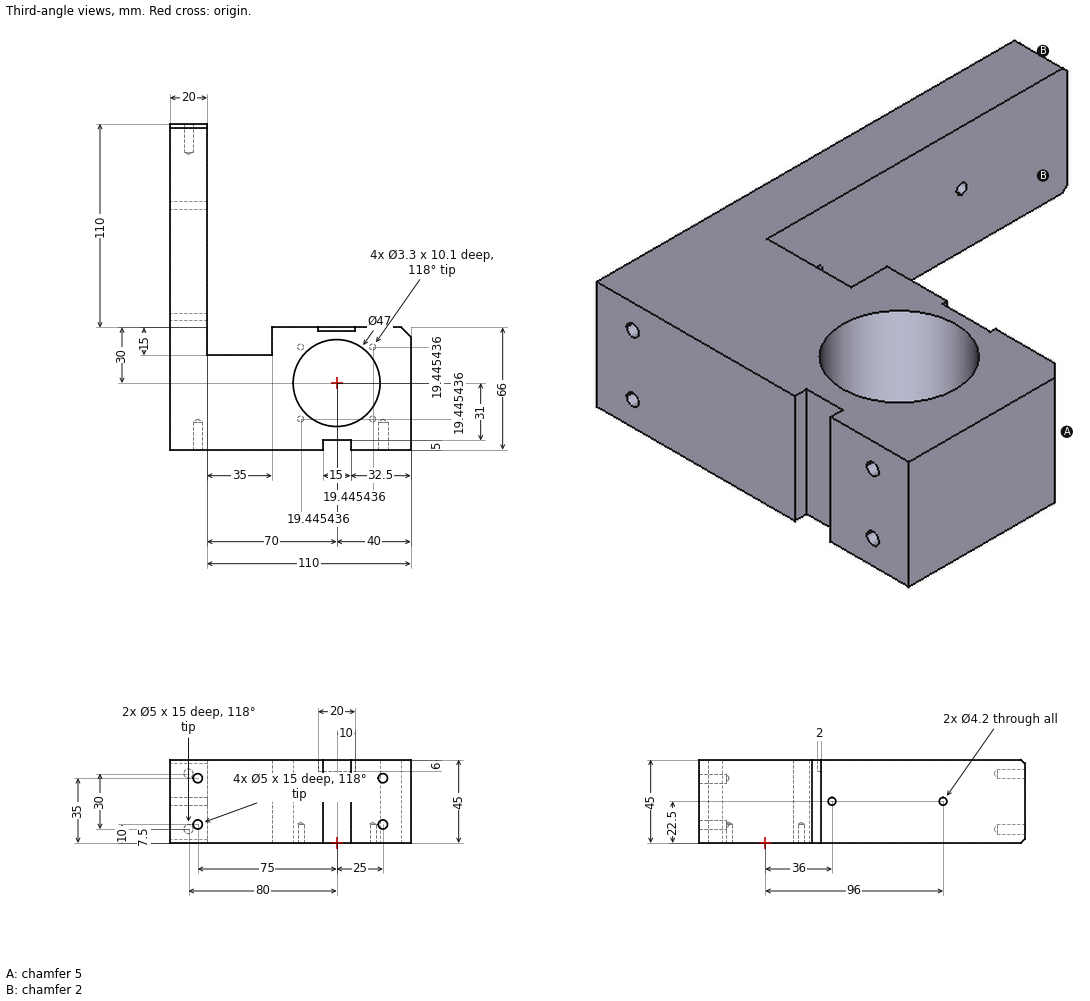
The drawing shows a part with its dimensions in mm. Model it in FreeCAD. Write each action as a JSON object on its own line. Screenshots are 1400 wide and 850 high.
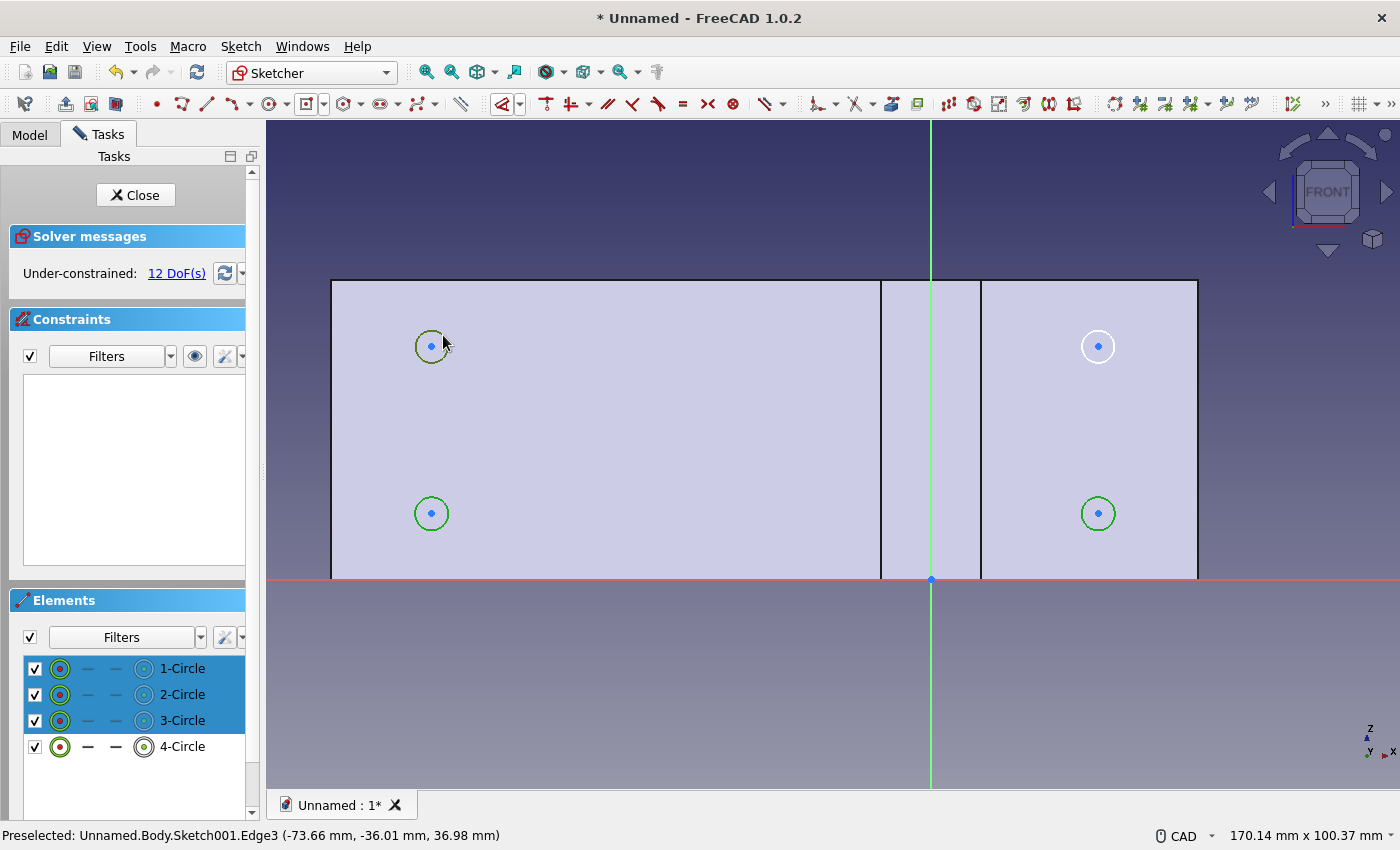
{"action": "left_click", "coordinate": [1110, 335]}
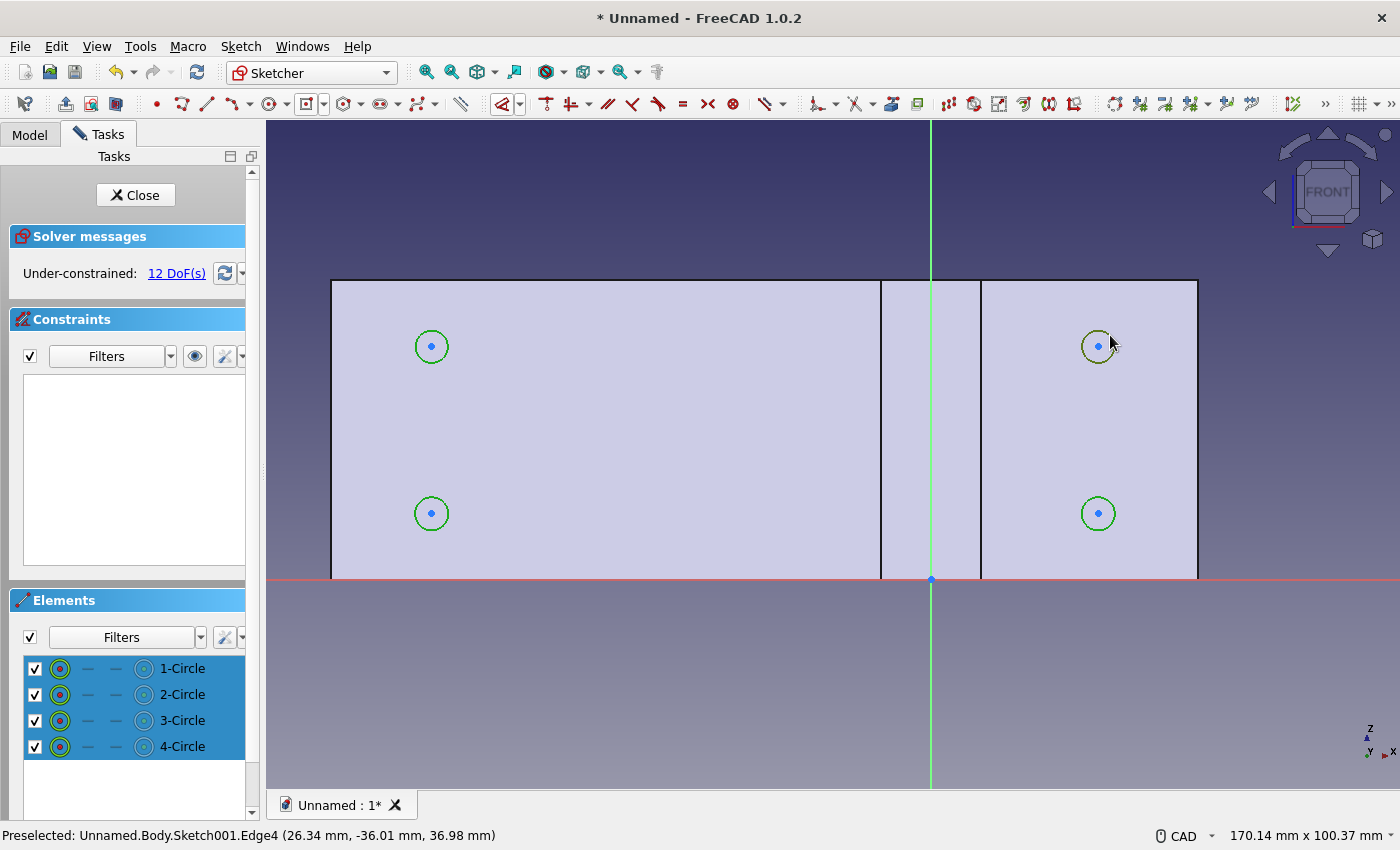
{"action": "key", "text": "e"}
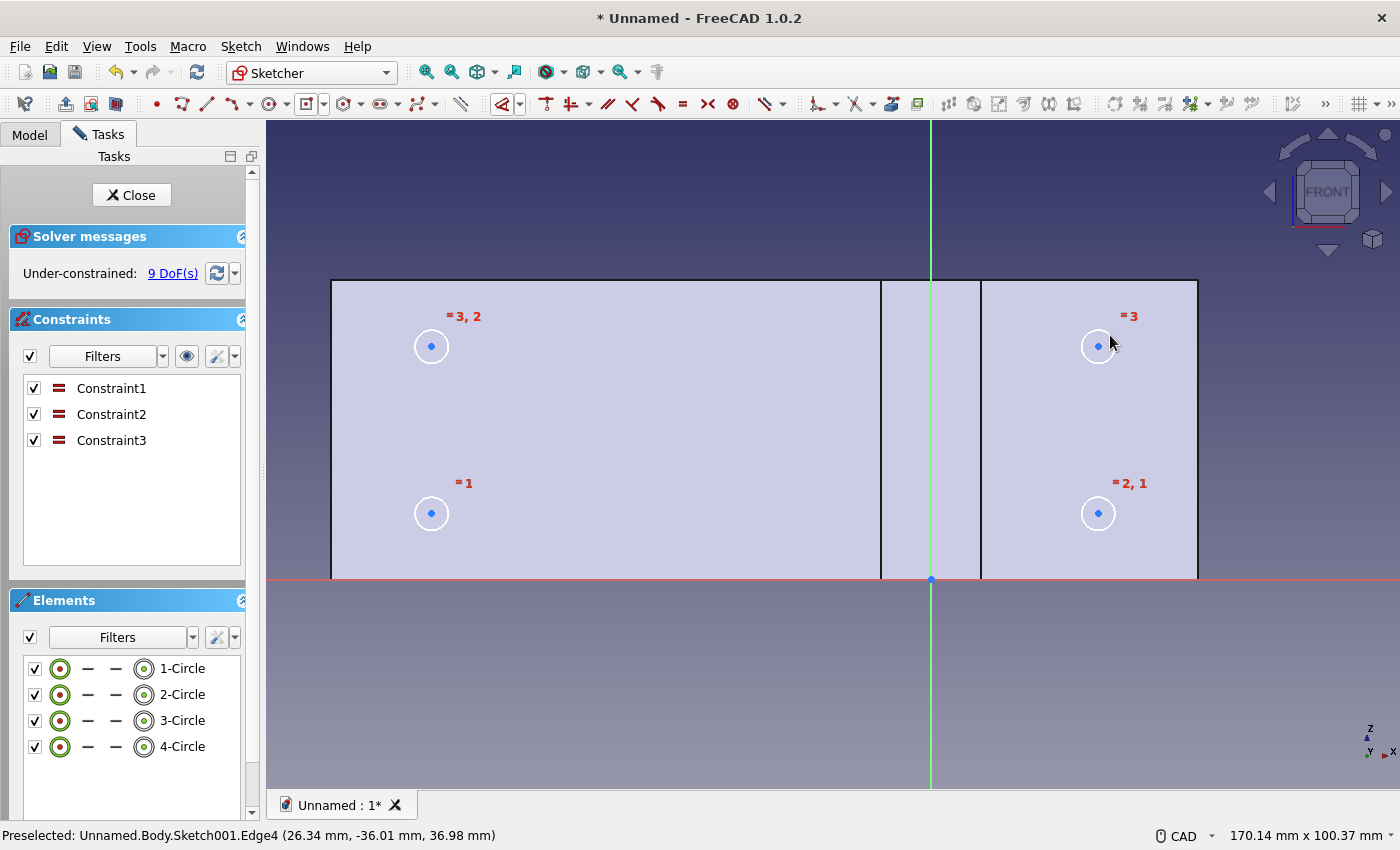
{"action": "left_click", "coordinate": [432, 514]}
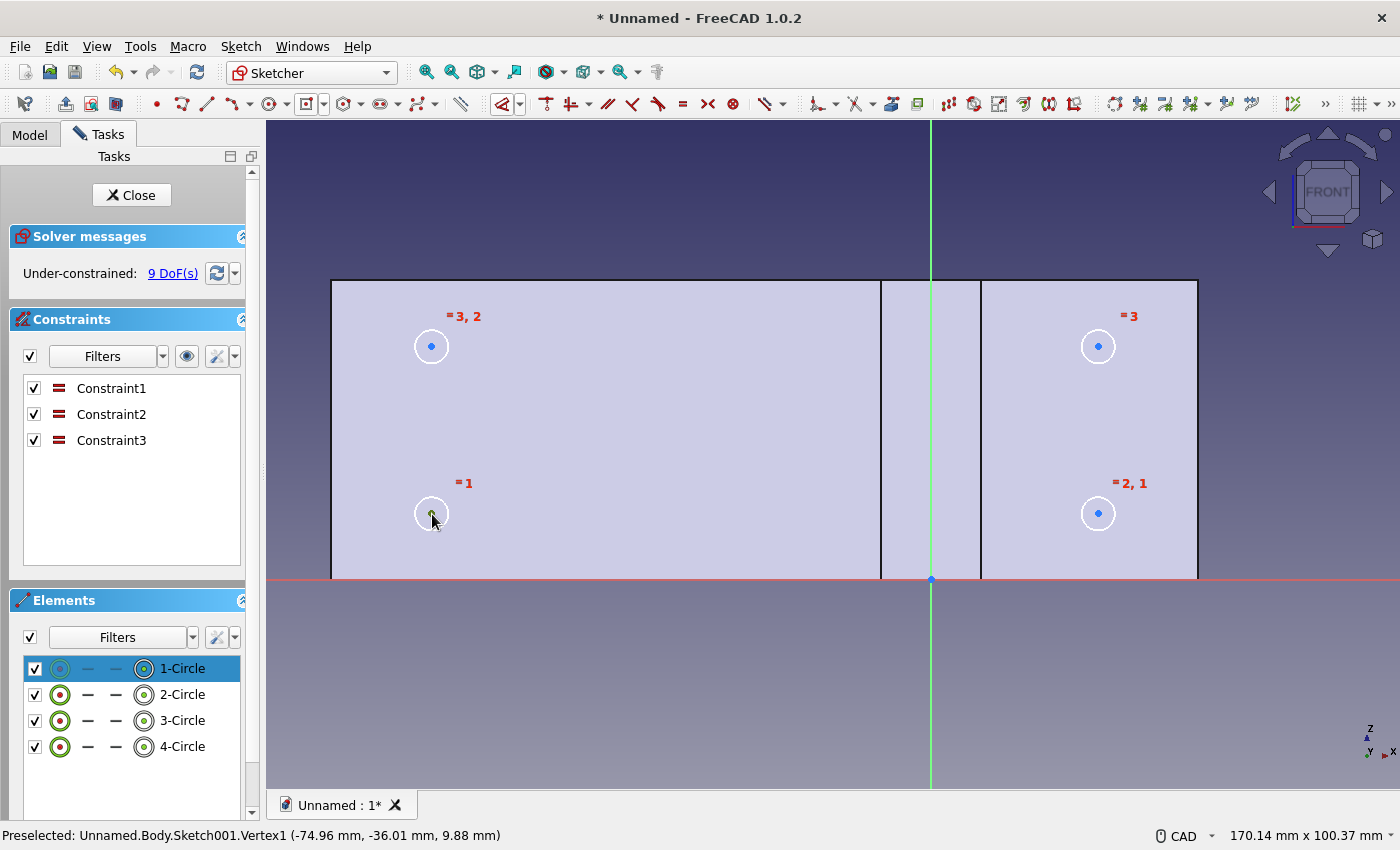
{"action": "left_click", "coordinate": [1098, 514]}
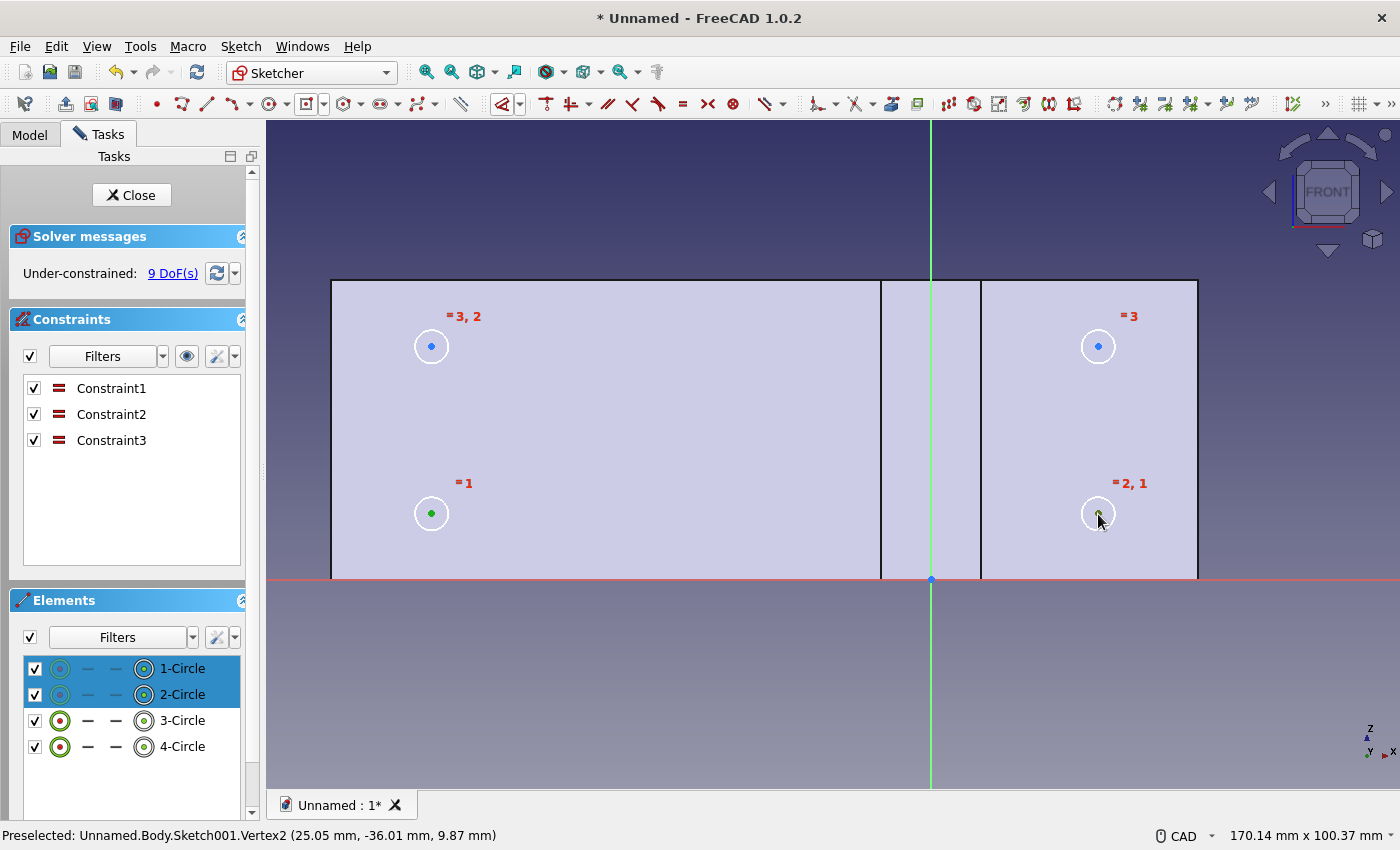
{"action": "key", "text": "h"}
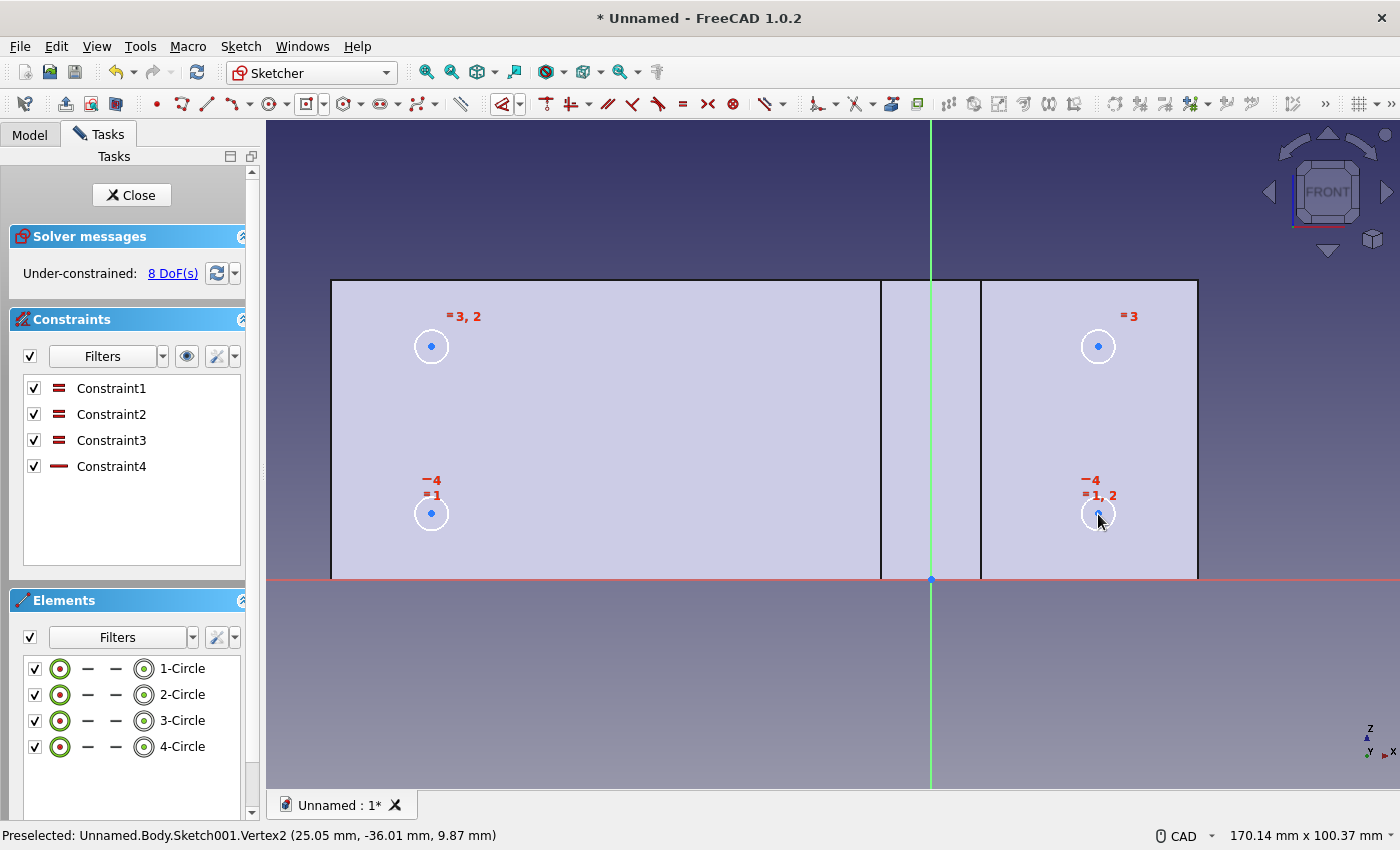
{"action": "left_click", "coordinate": [432, 514]}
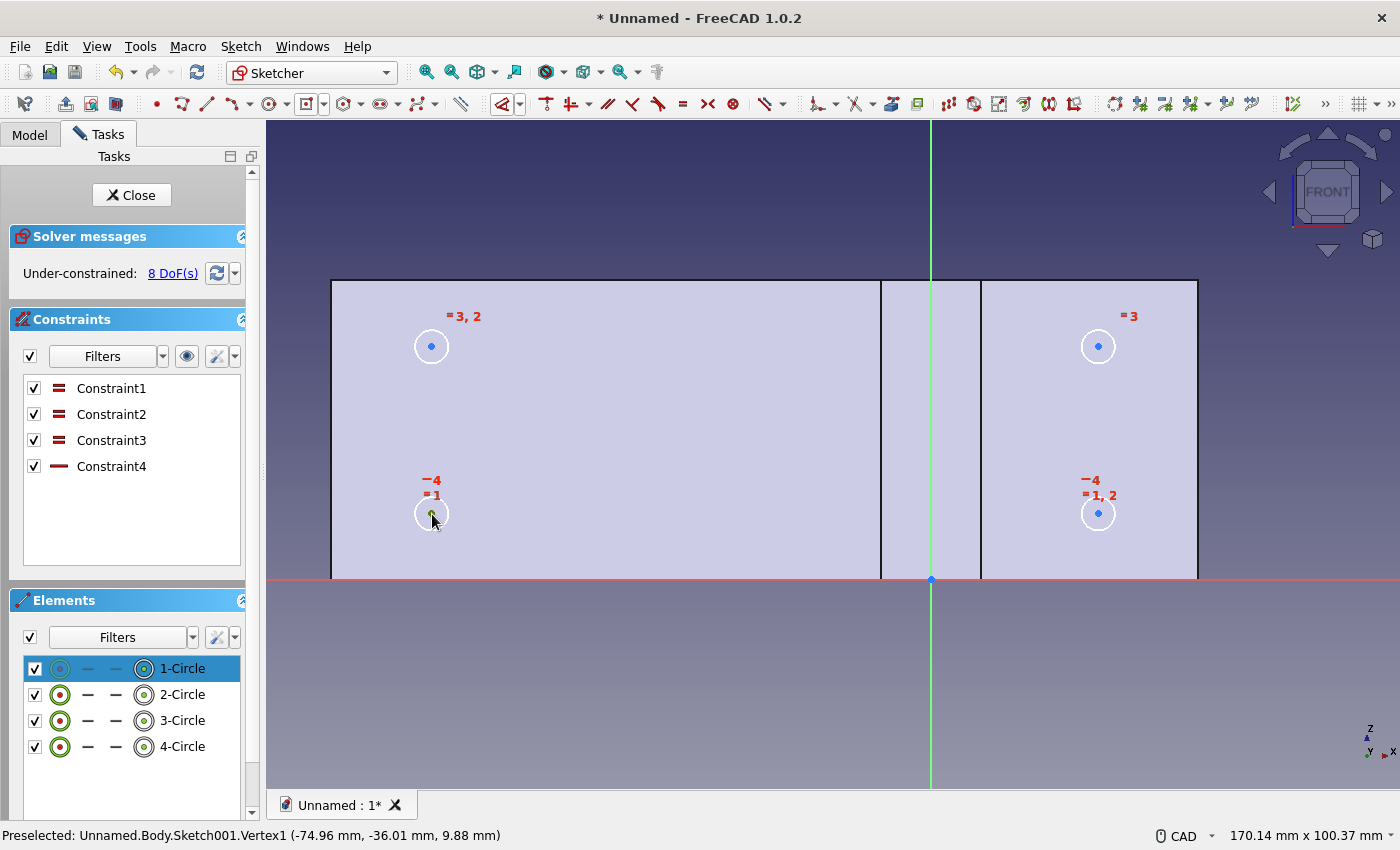
{"action": "left_click", "coordinate": [432, 347]}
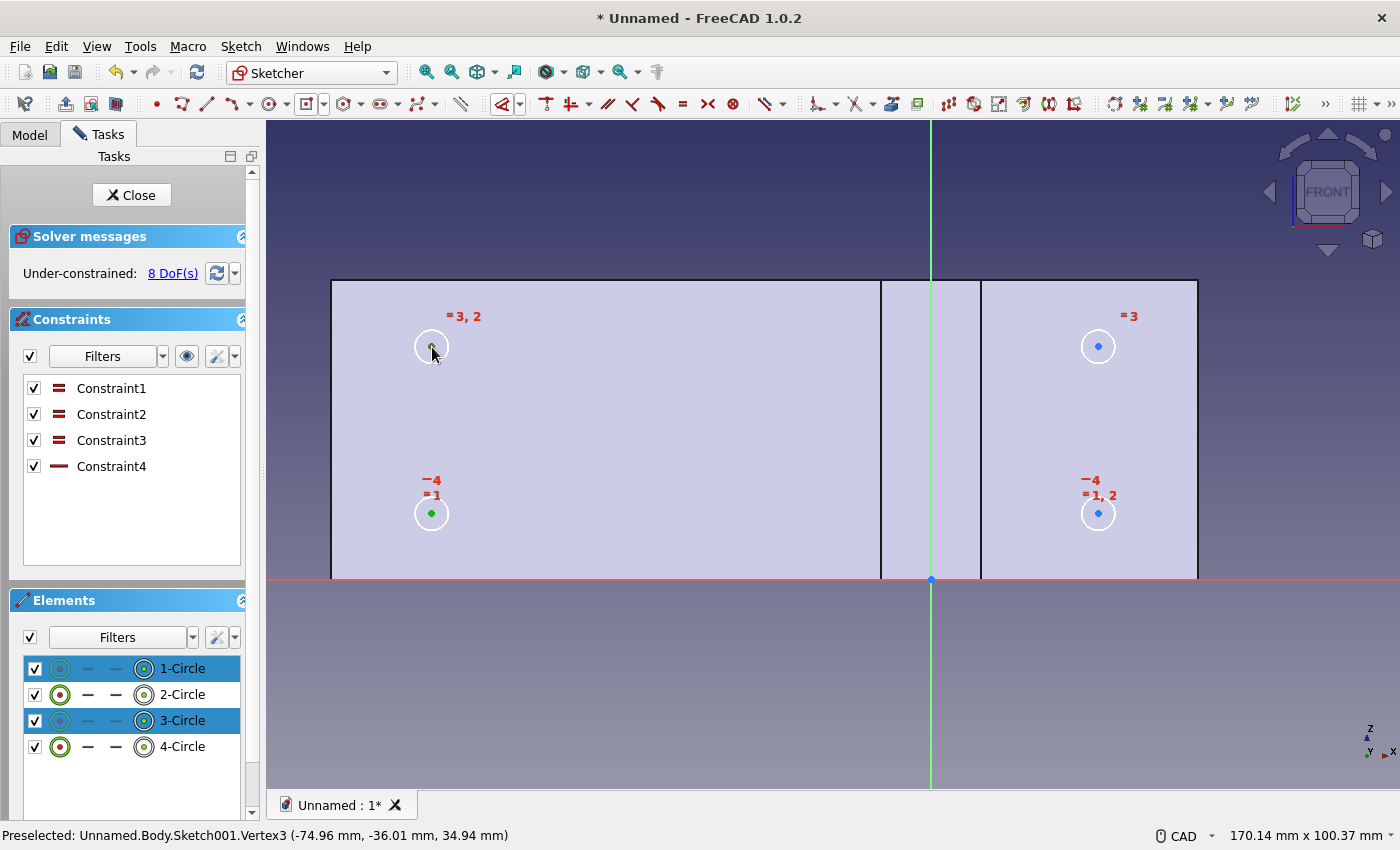
{"action": "left_click", "coordinate": [588, 104]}